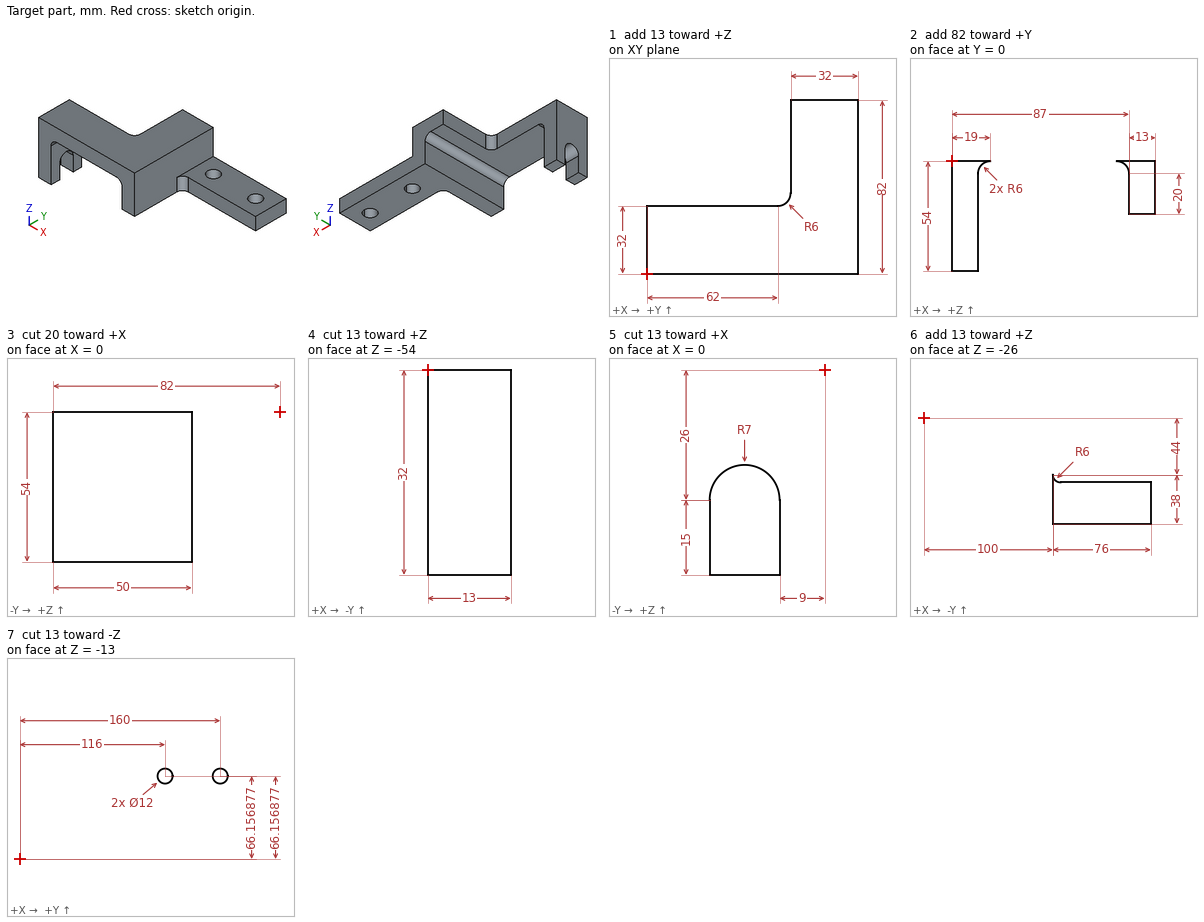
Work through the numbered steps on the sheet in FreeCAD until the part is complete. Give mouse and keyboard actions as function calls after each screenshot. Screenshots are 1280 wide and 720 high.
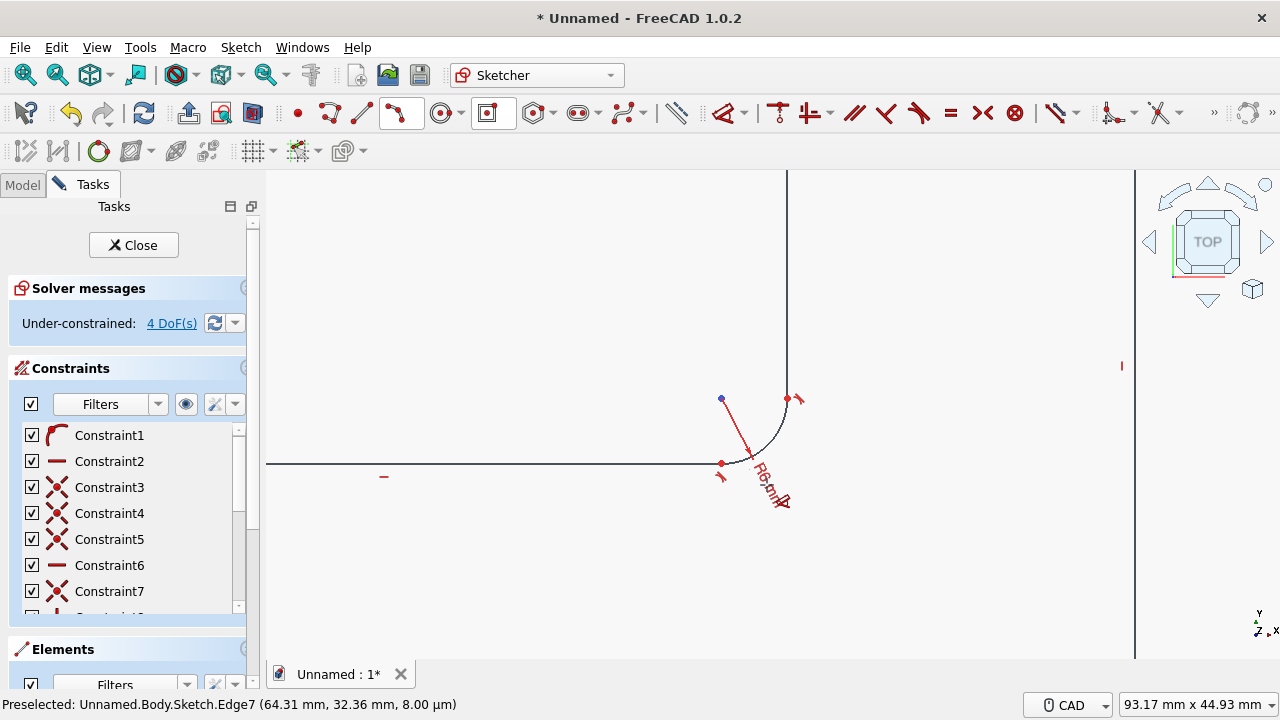
click(520, 464)
click(508, 498)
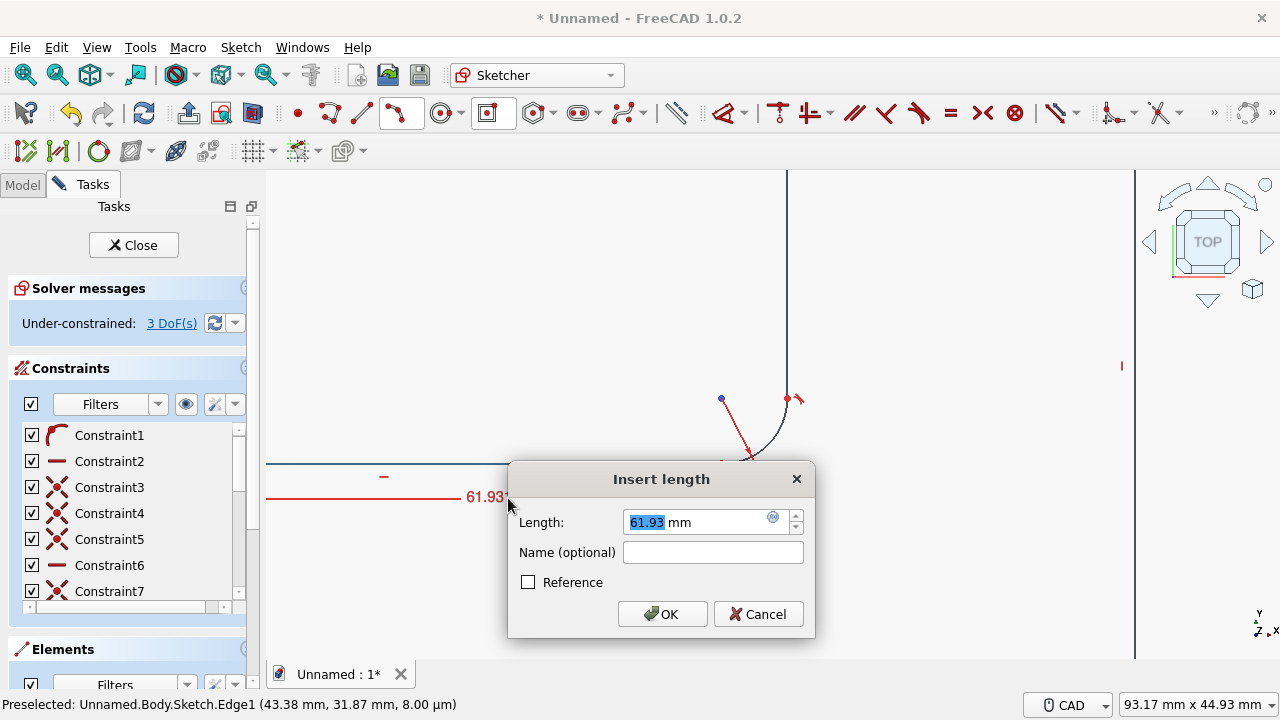
text(62)
key(Return)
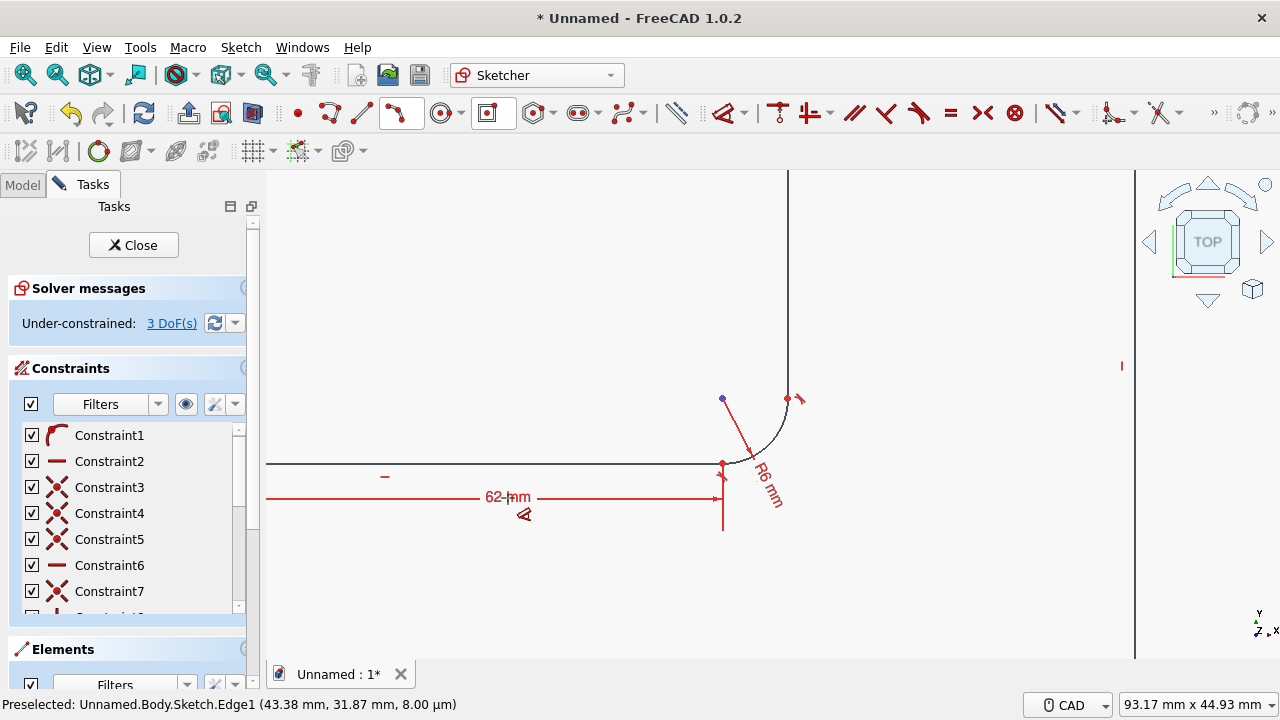
scroll(770, 444, down, 5)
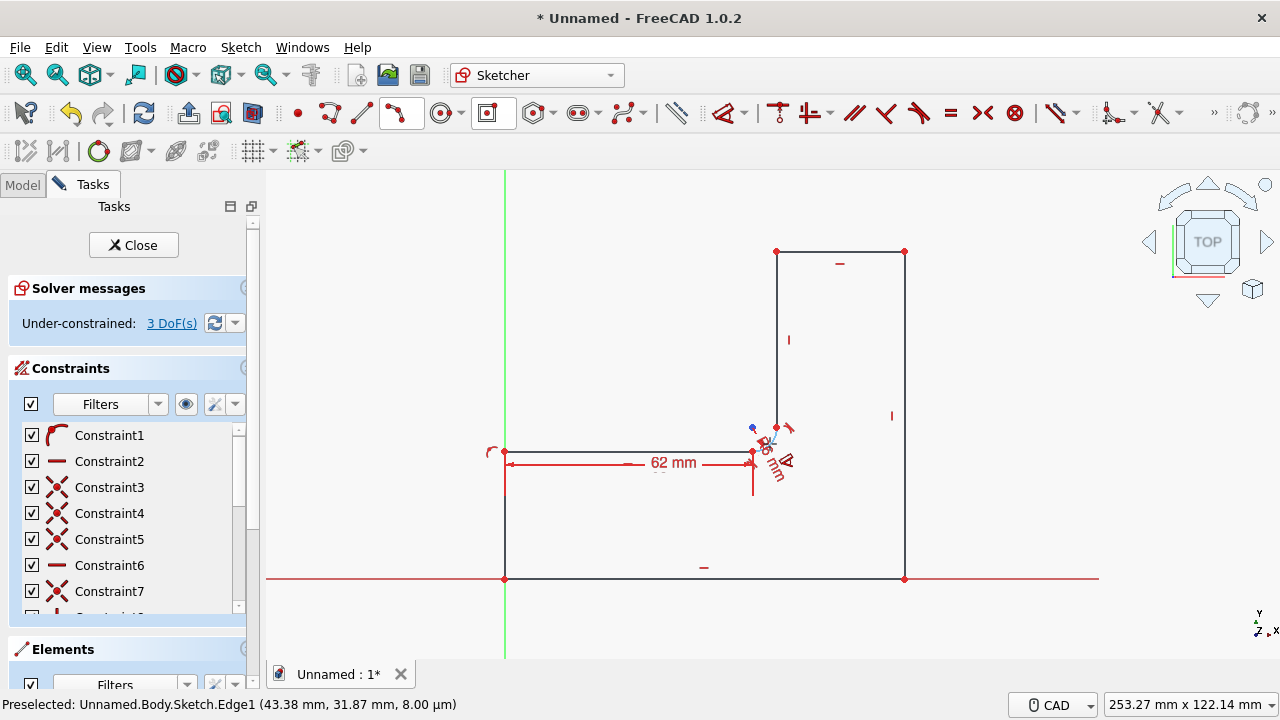
click(505, 490)
click(471, 515)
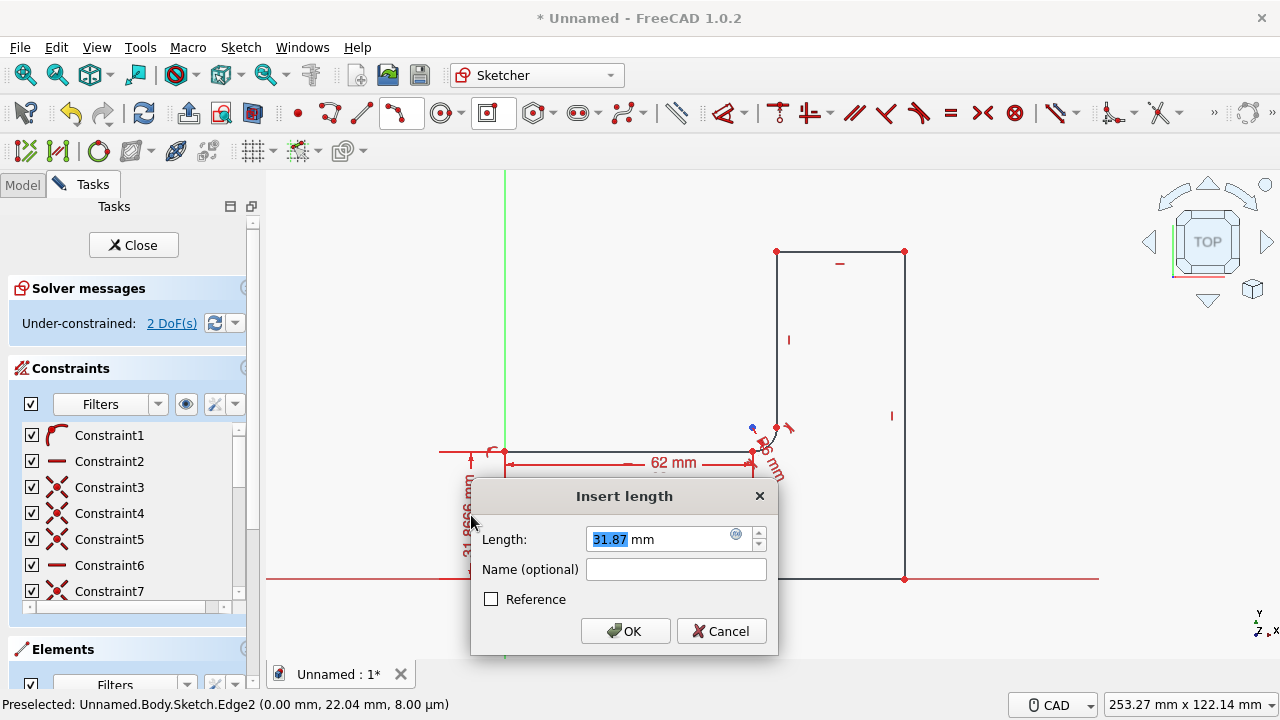
text(32)
key(Return)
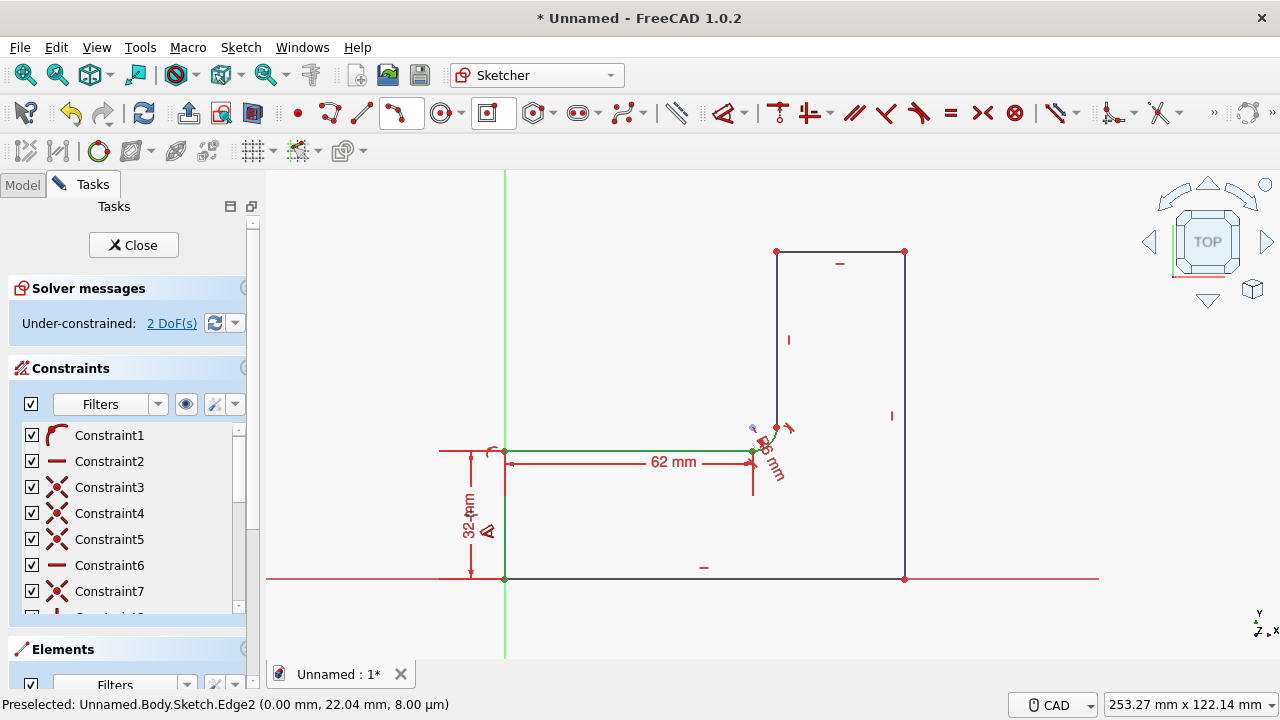
click(905, 481)
click(939, 415)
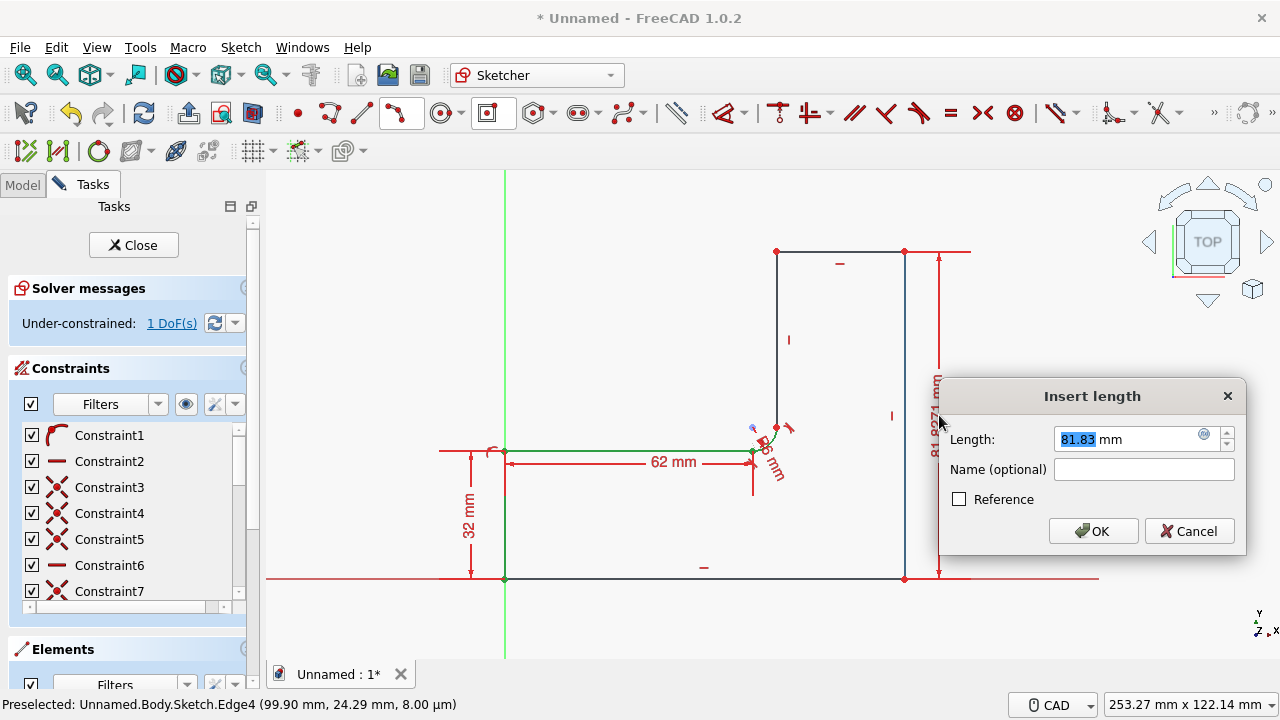
text(82)
key(Return)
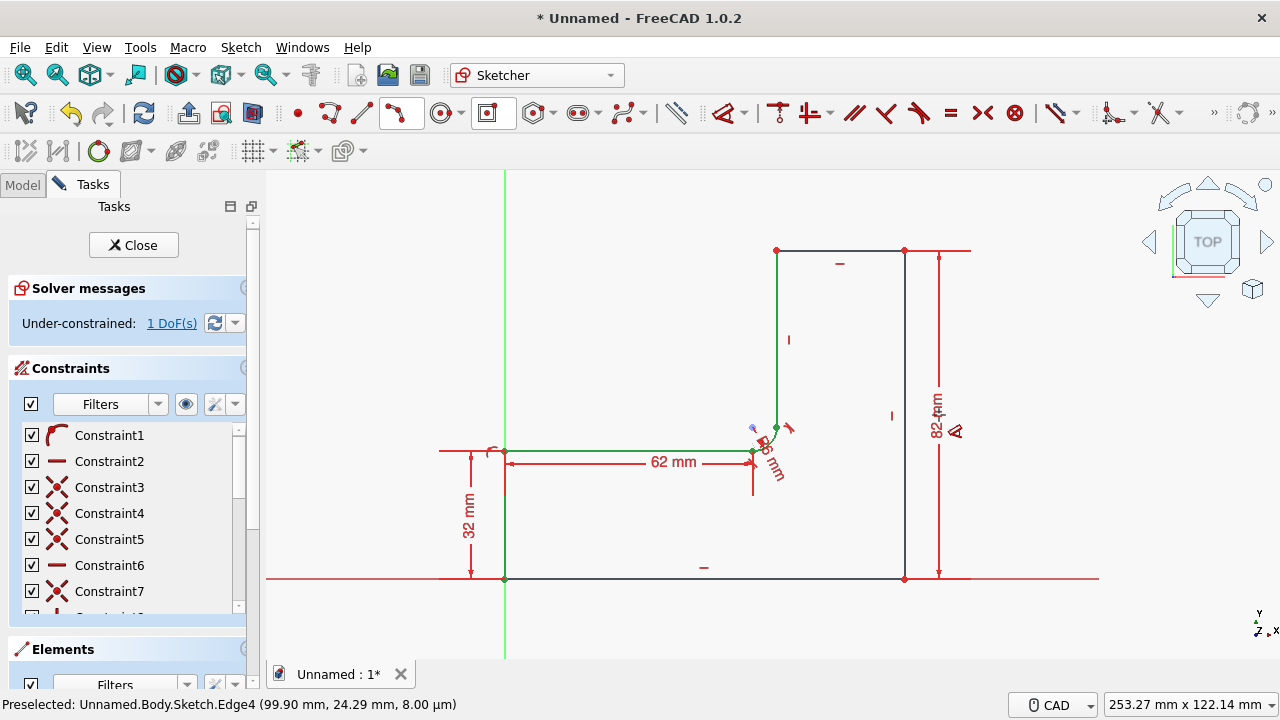
click(866, 251)
click(841, 217)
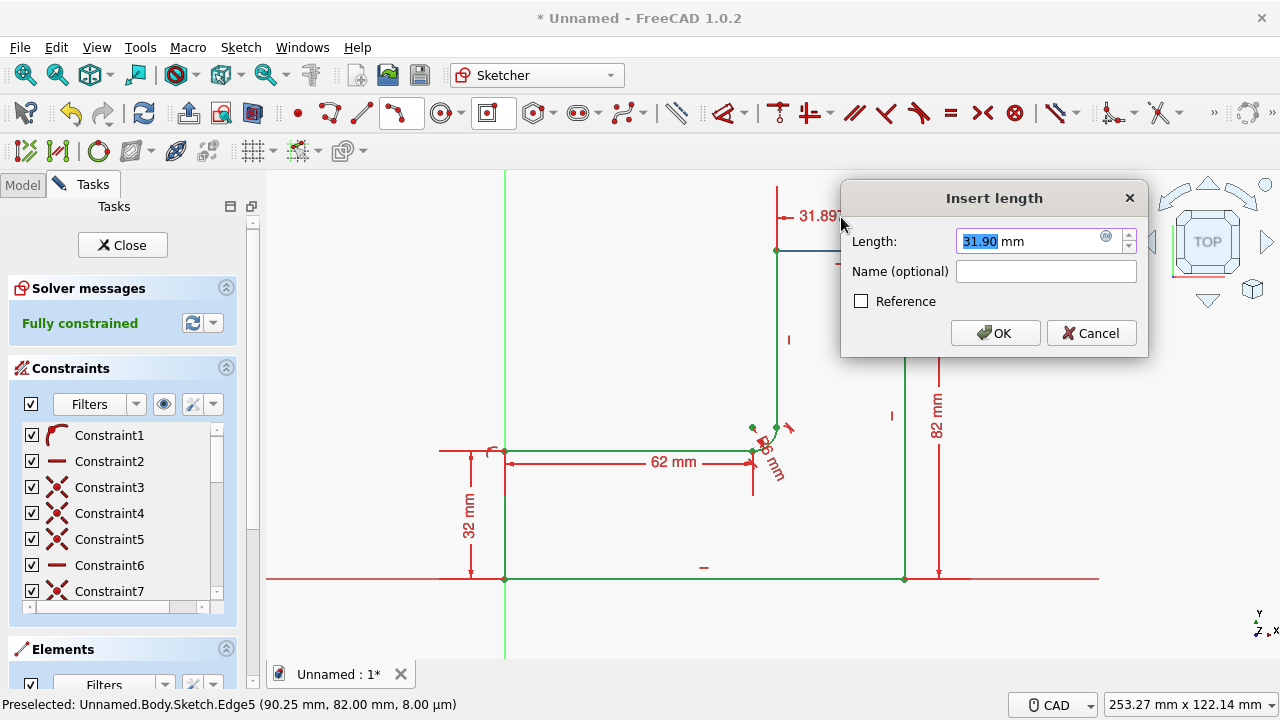
text(32)
key(Return)
key(Escape)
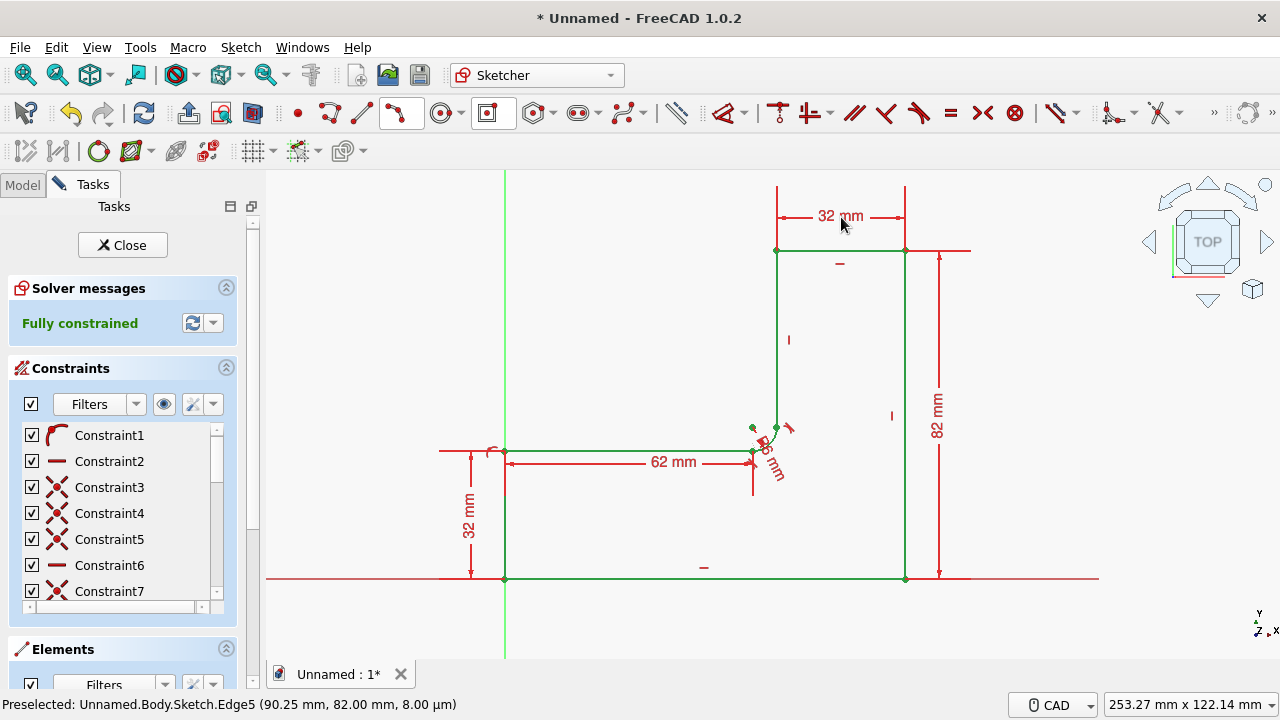
click(123, 245)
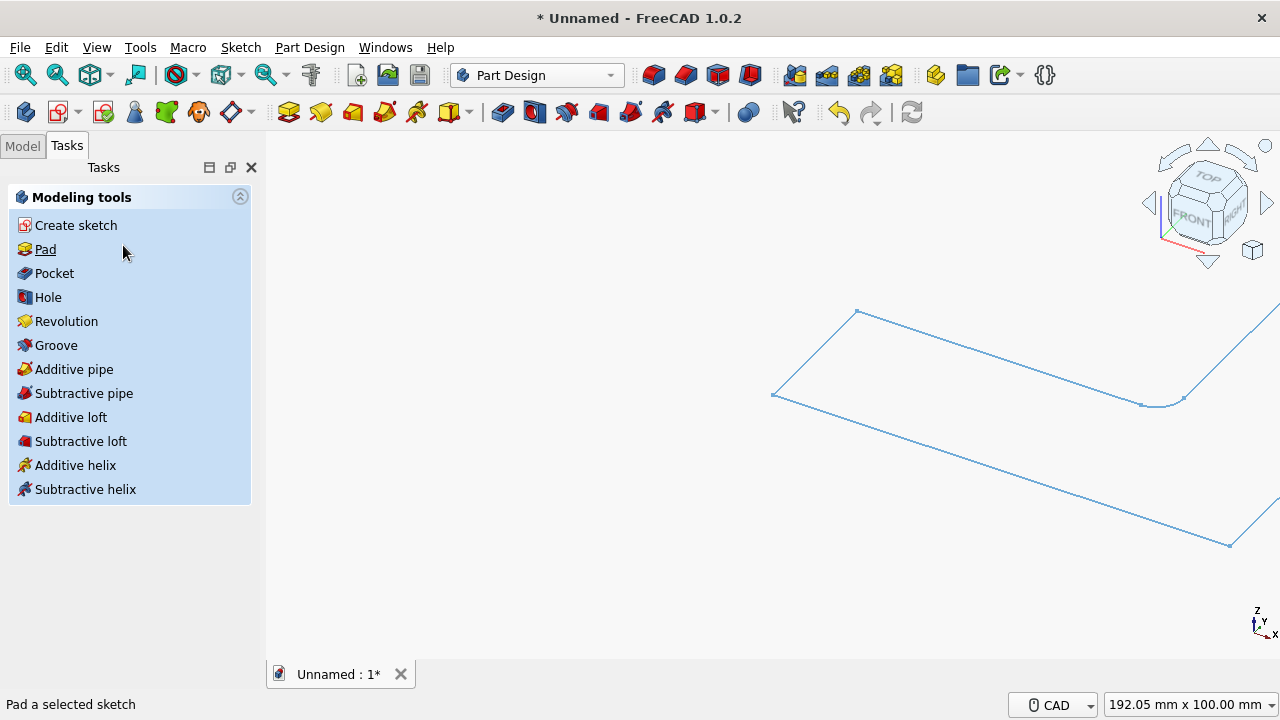
click(290, 112)